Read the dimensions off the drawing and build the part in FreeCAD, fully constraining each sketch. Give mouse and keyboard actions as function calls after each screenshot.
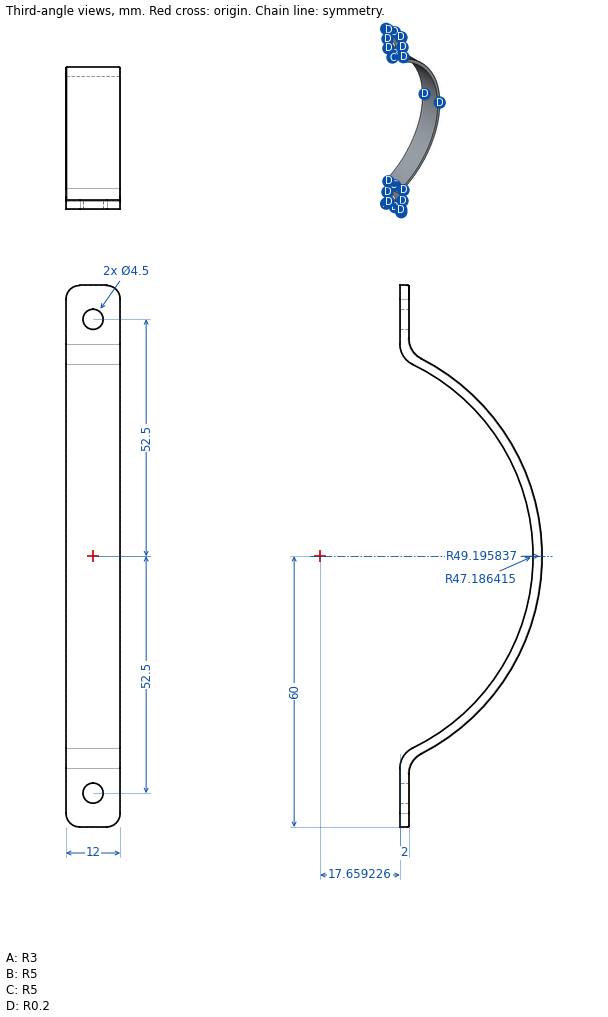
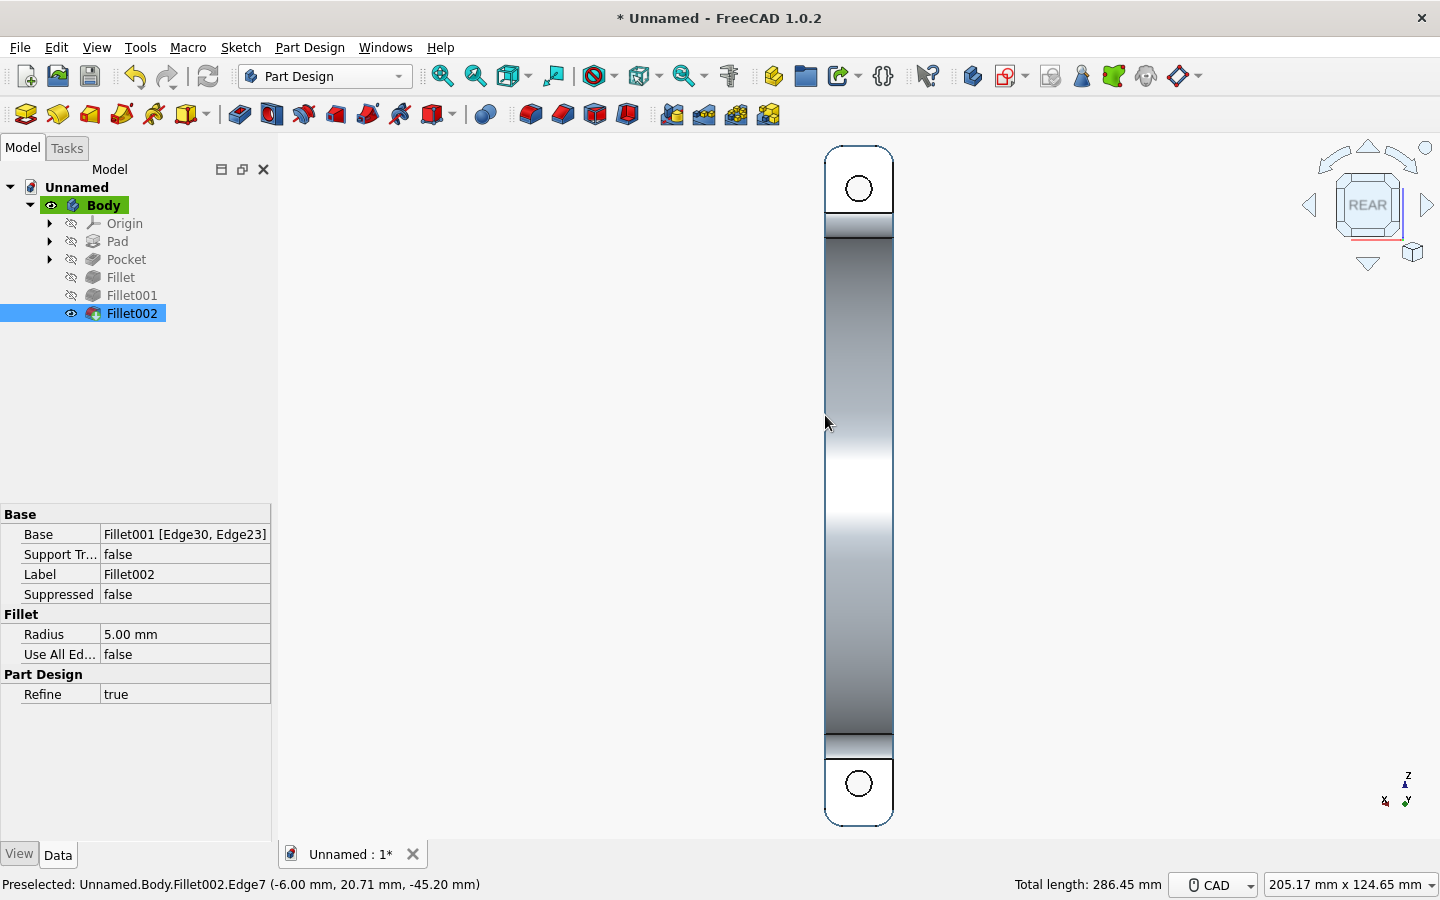
click(893, 783, ctrl)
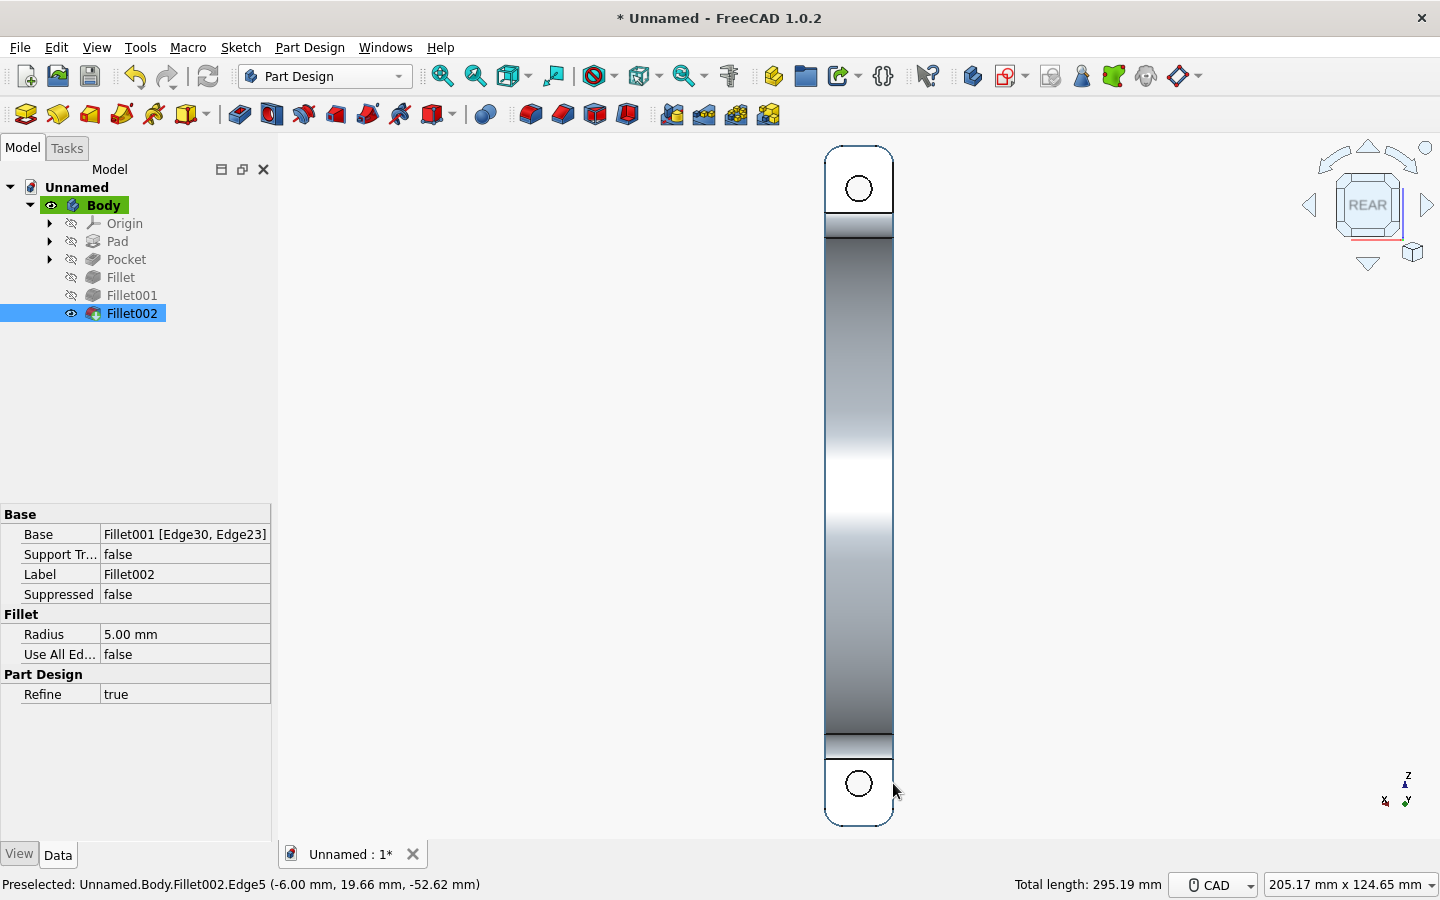
click(893, 187, ctrl)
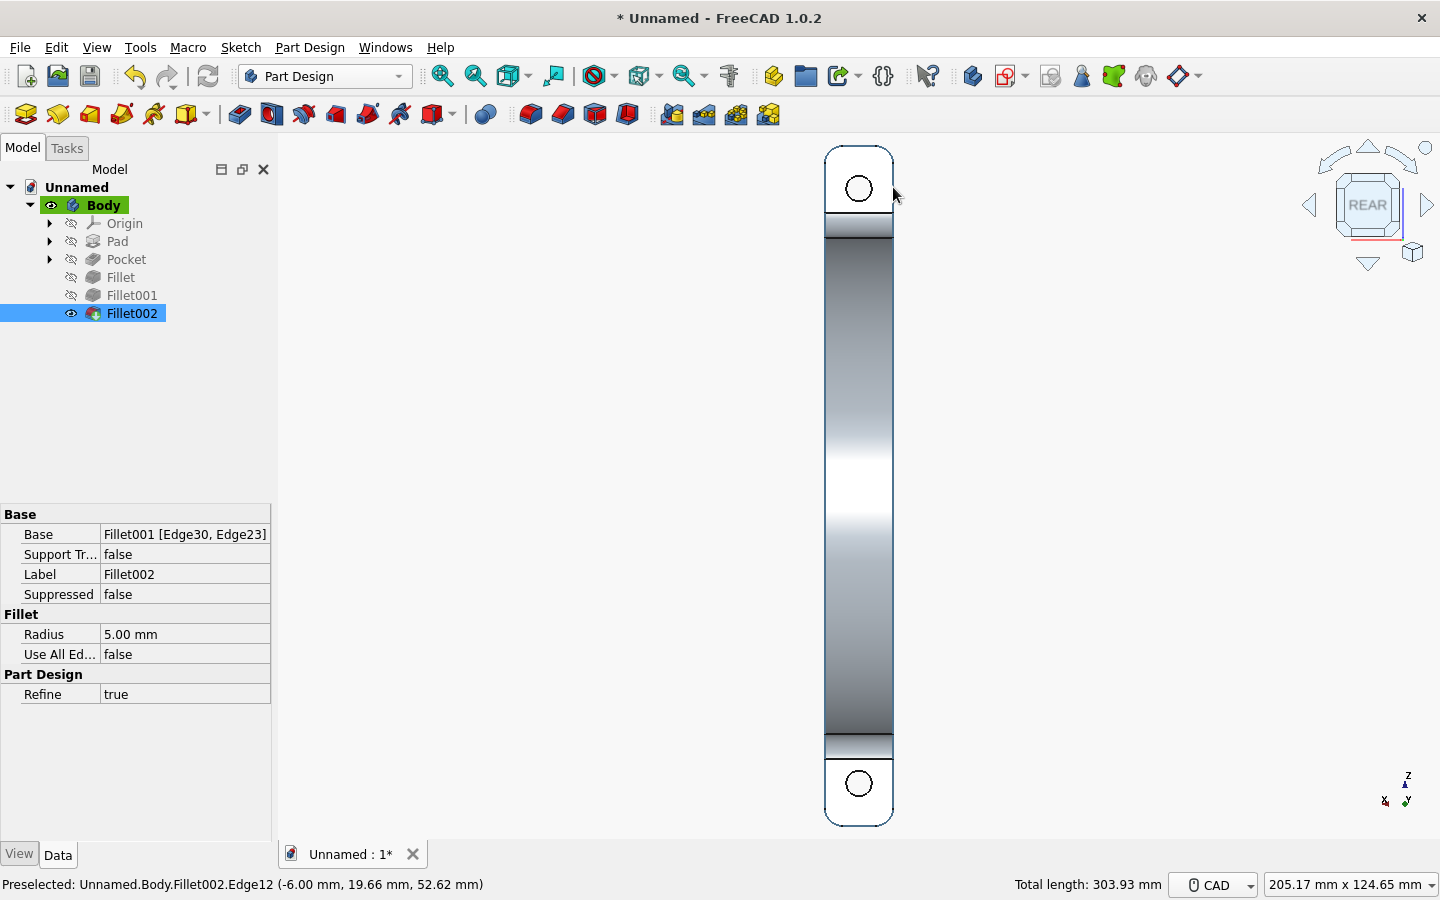
click(532, 114)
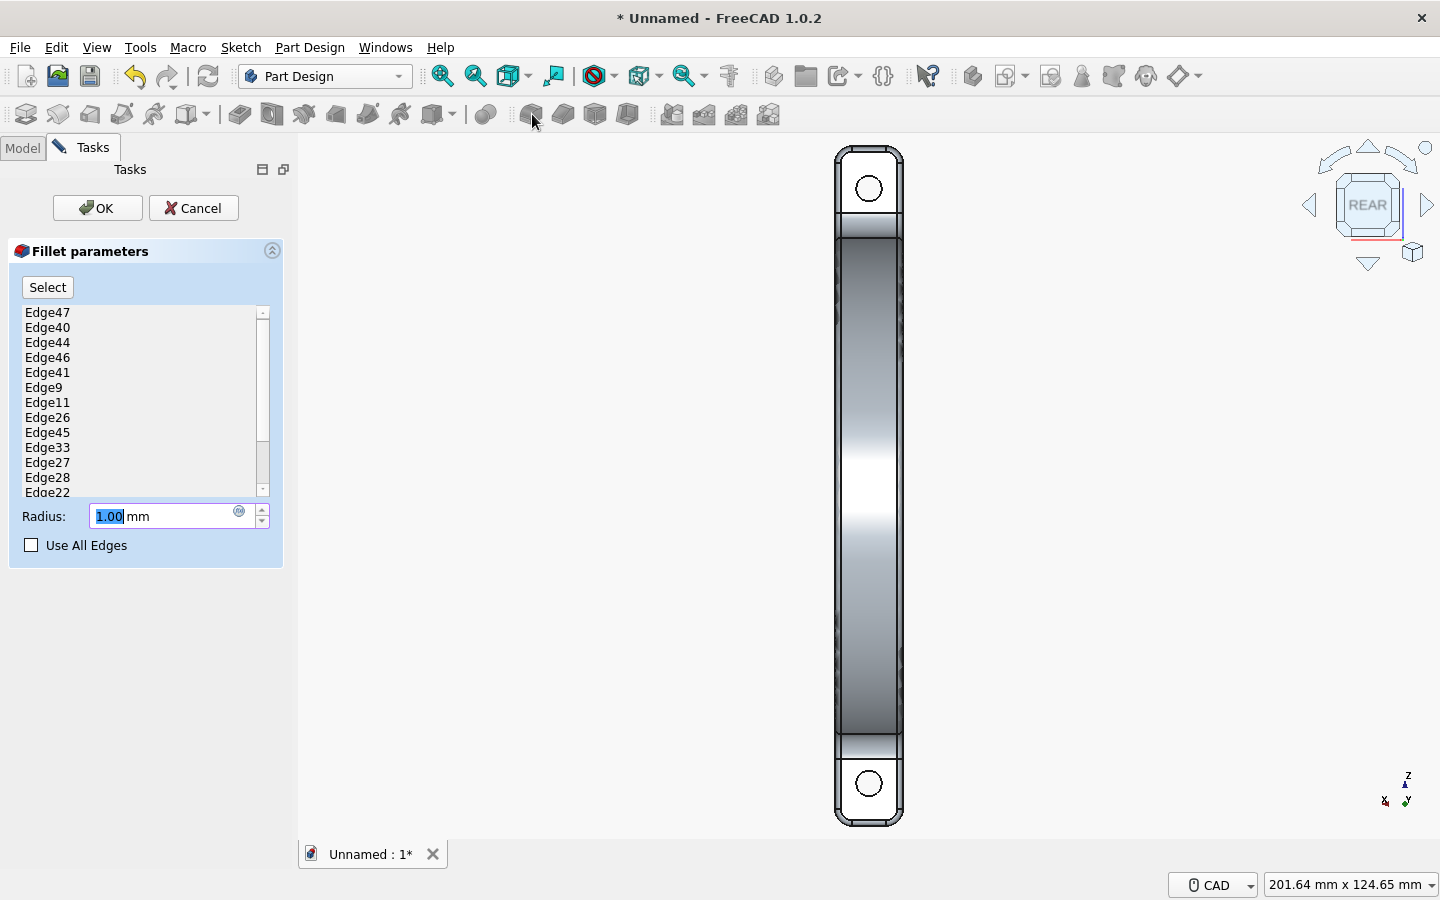
text(0.2)
key(Tab)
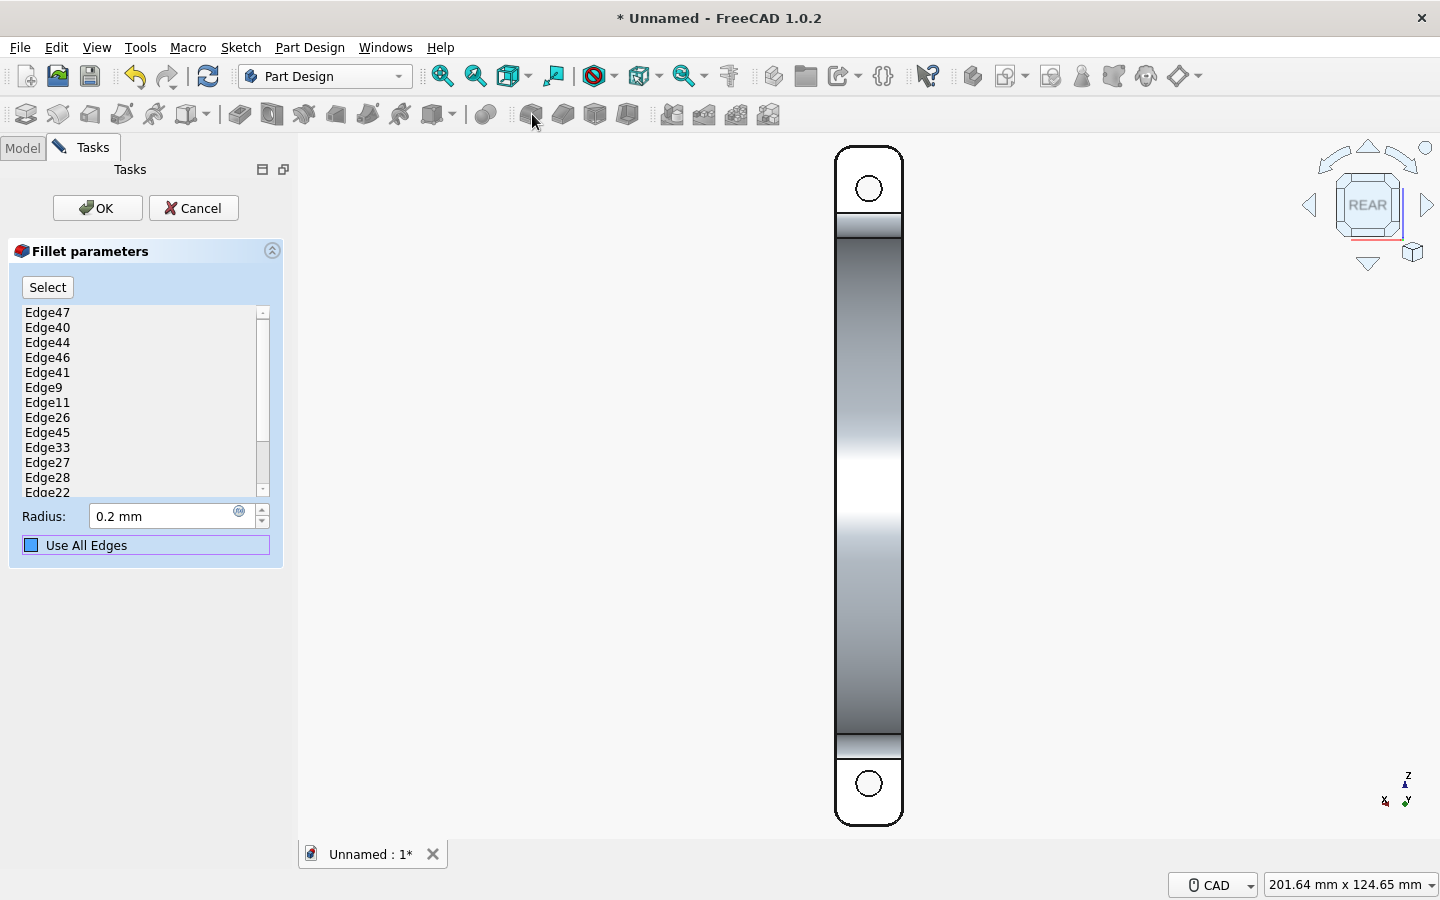
click(98, 208)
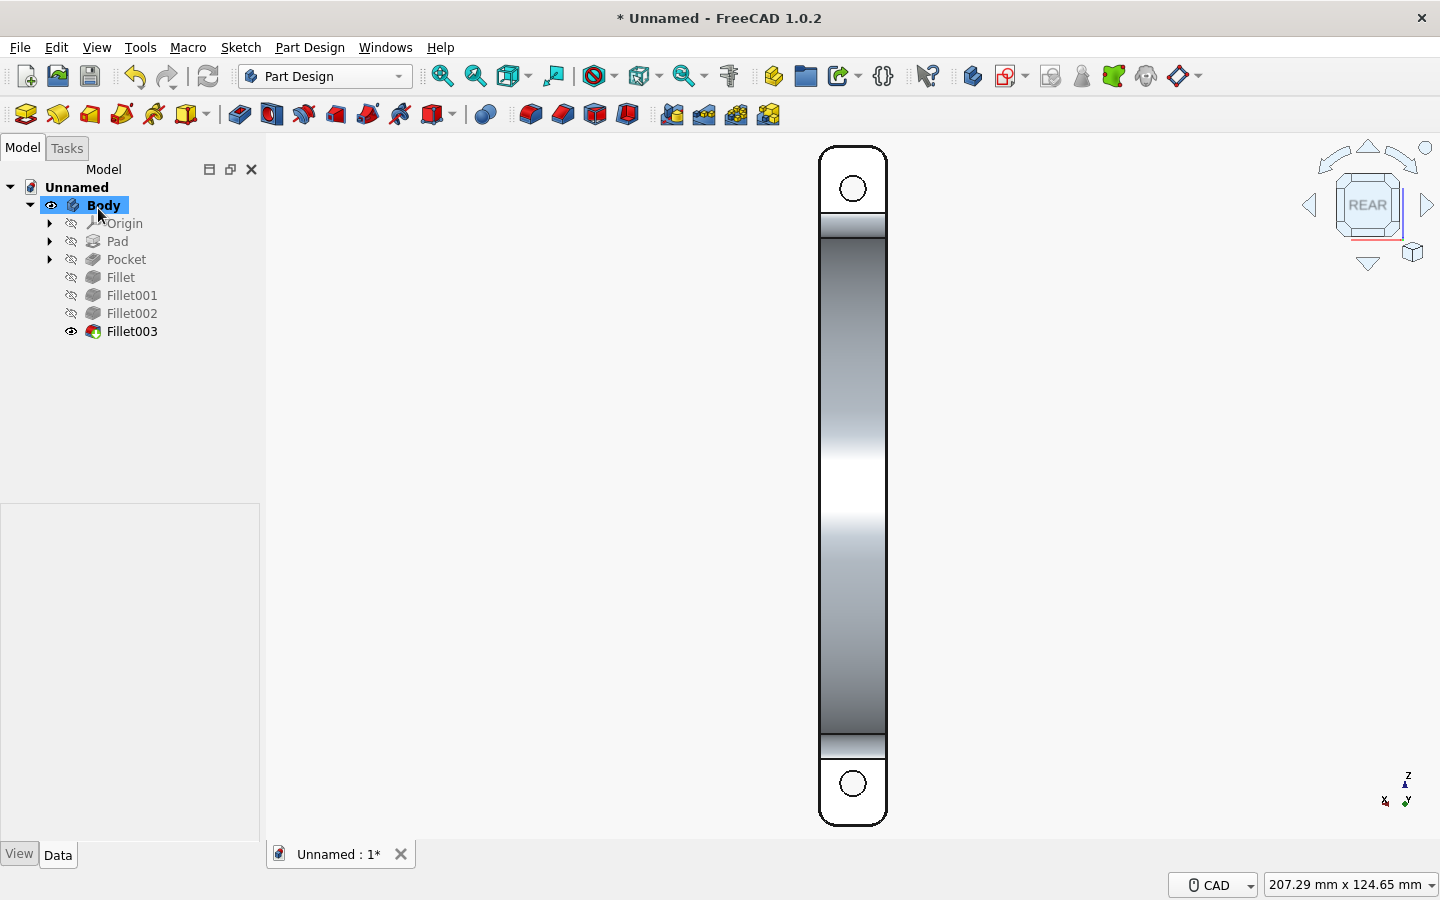
key(0)